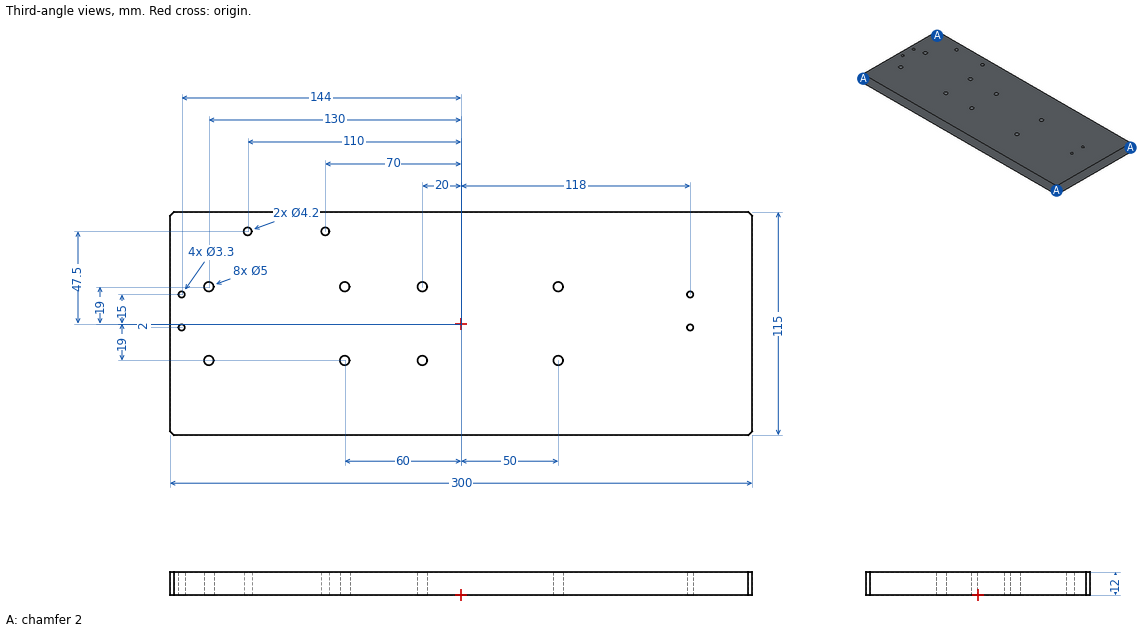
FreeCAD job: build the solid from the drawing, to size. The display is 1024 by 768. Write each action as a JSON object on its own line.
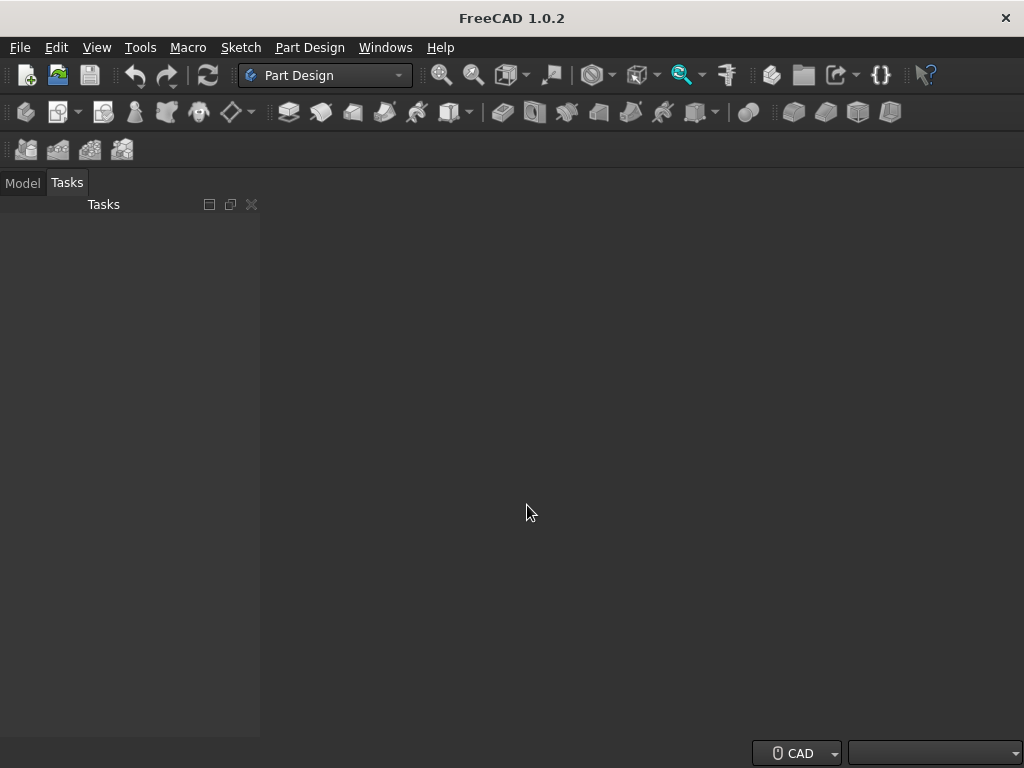
{"action": "left_click", "coordinate": [26, 76]}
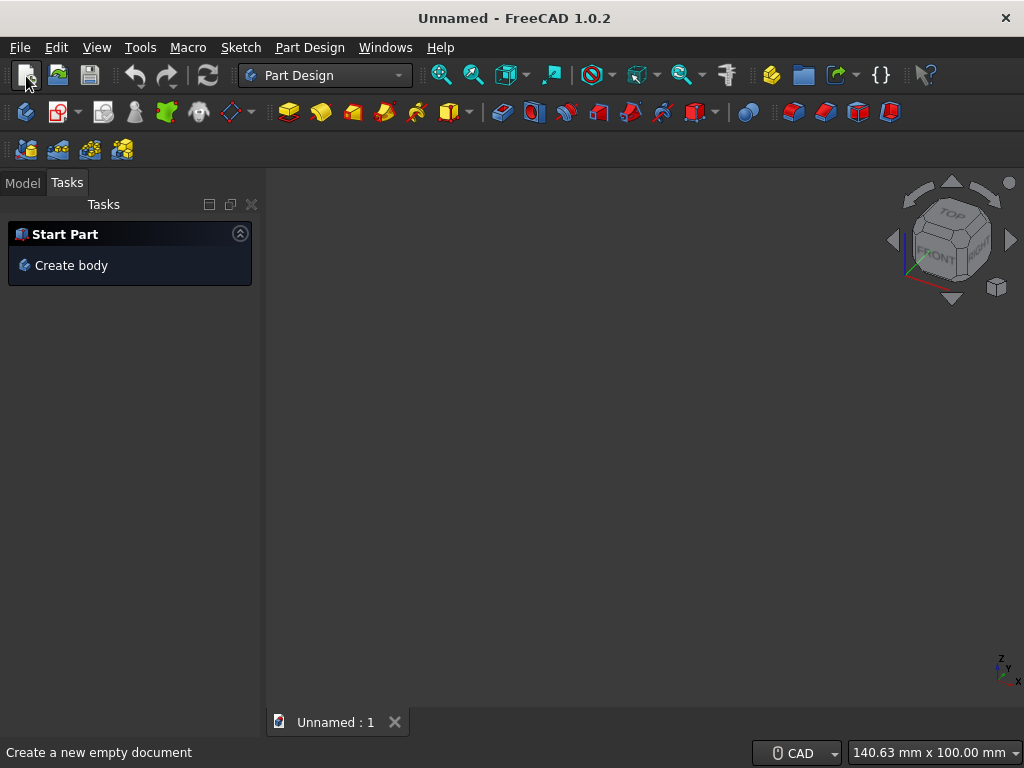
{"action": "left_click", "coordinate": [58, 112]}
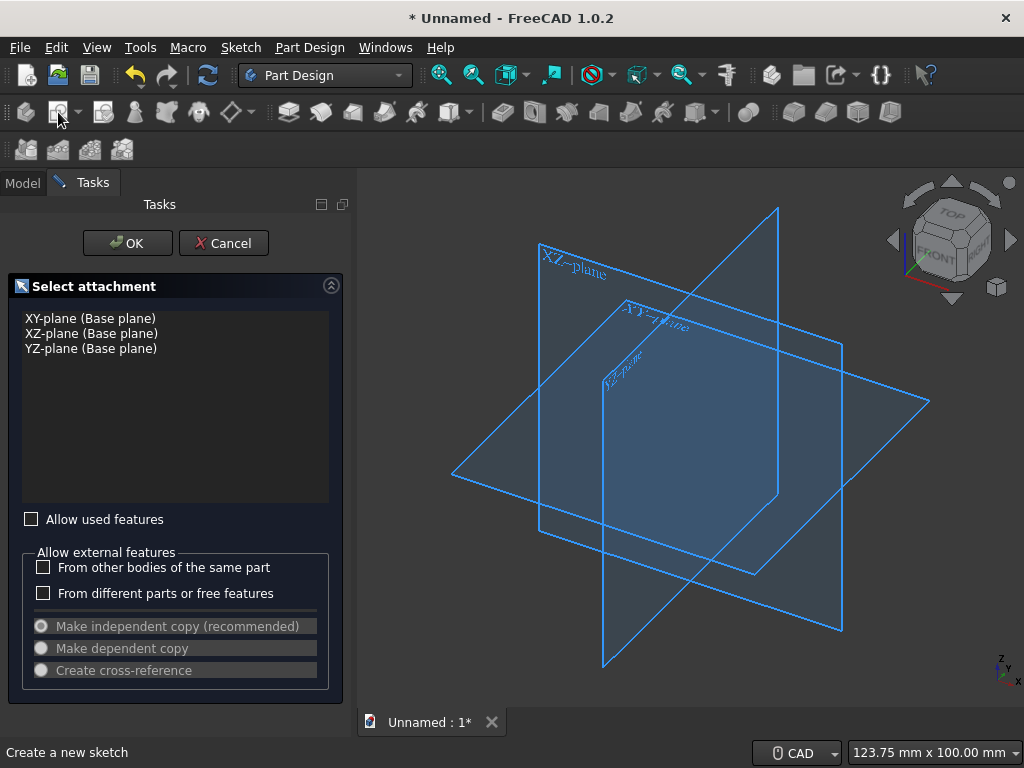
{"action": "left_click", "coordinate": [82, 318]}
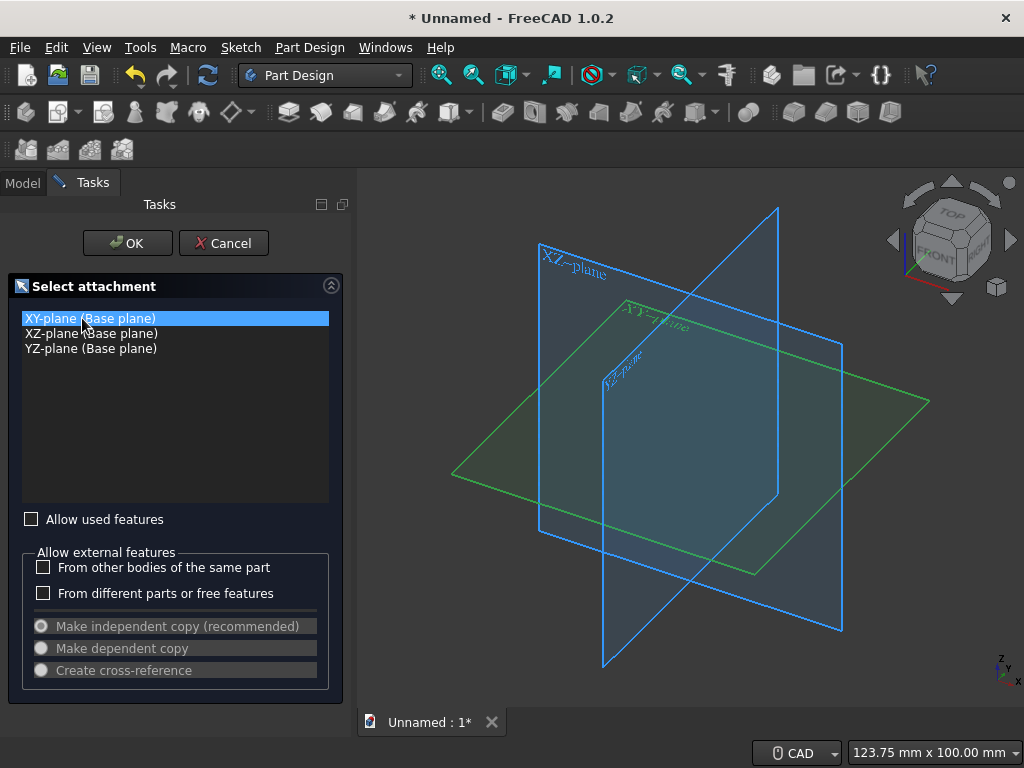
{"action": "left_click", "coordinate": [128, 243]}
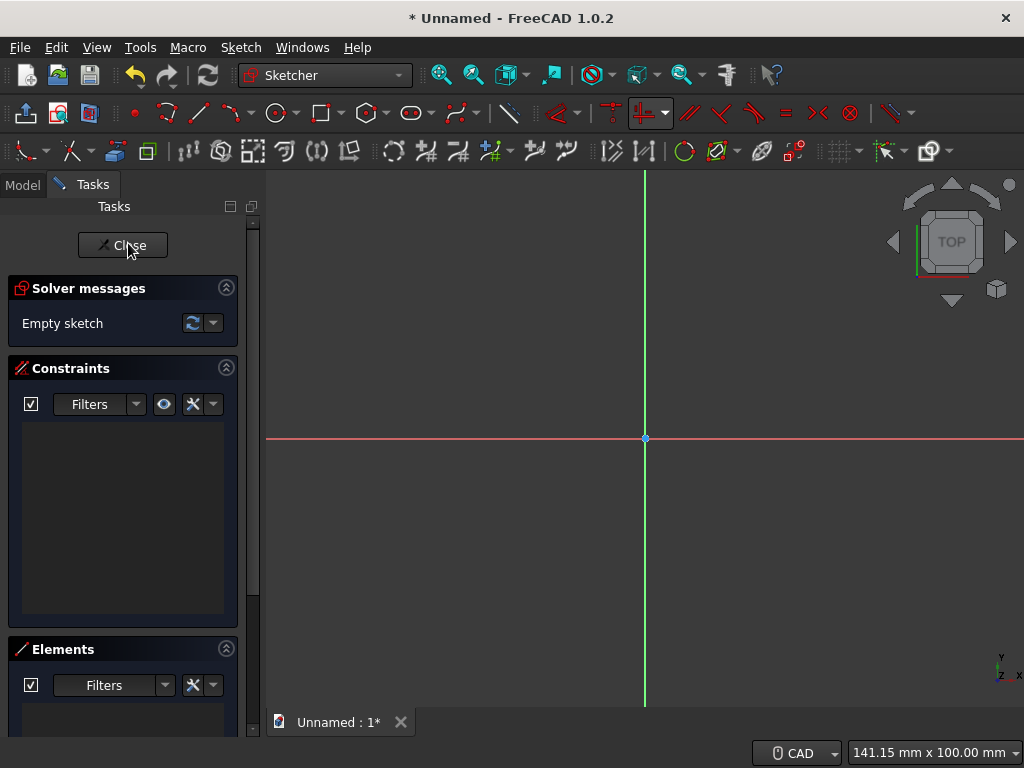
{"action": "scroll", "coordinate": [554, 438], "scroll_direction": "down", "scroll_amount": 7}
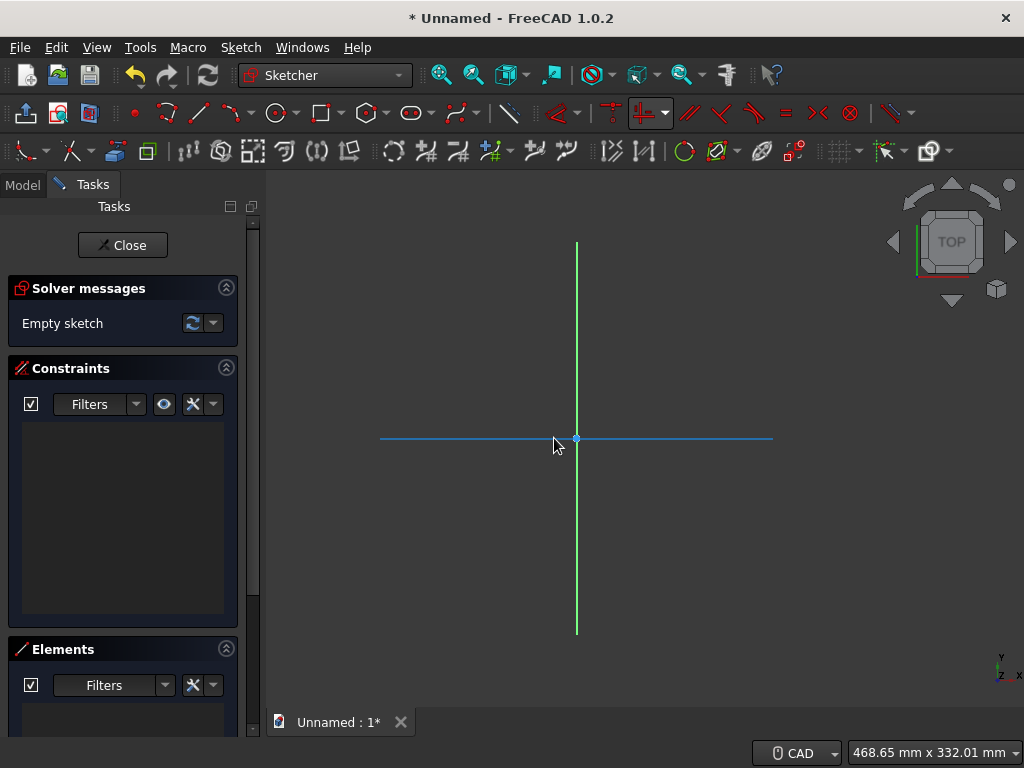
{"action": "key", "text": "g v"}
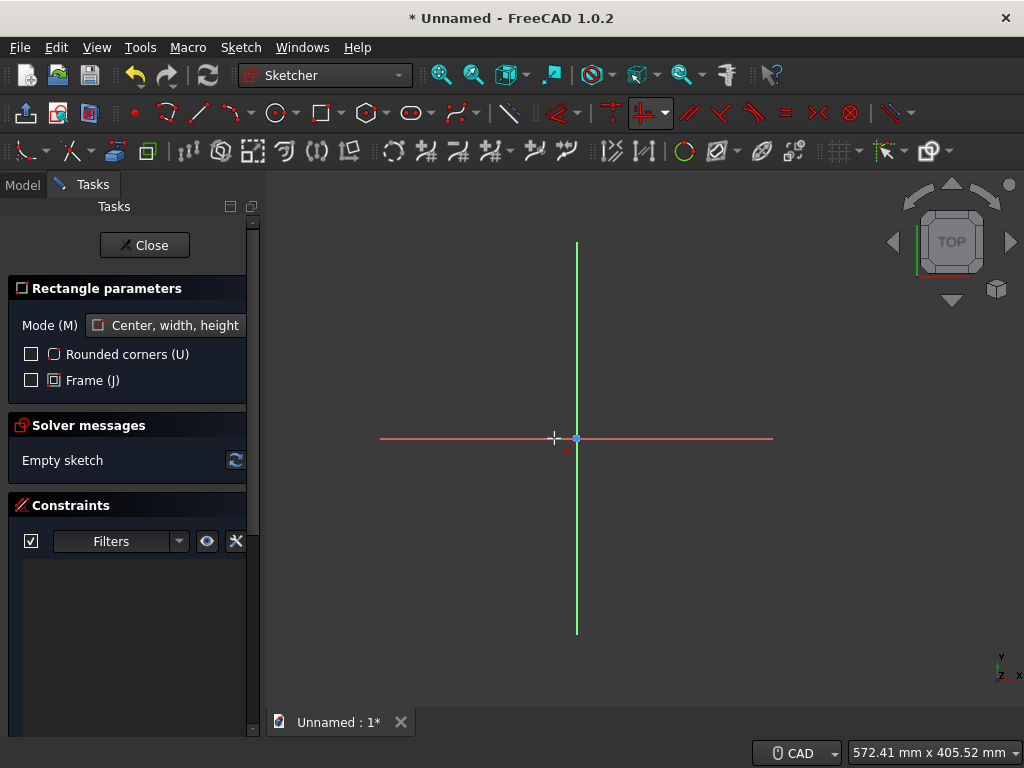
{"action": "left_click", "coordinate": [577, 438]}
{"action": "mouse_move", "coordinate": [775, 362]}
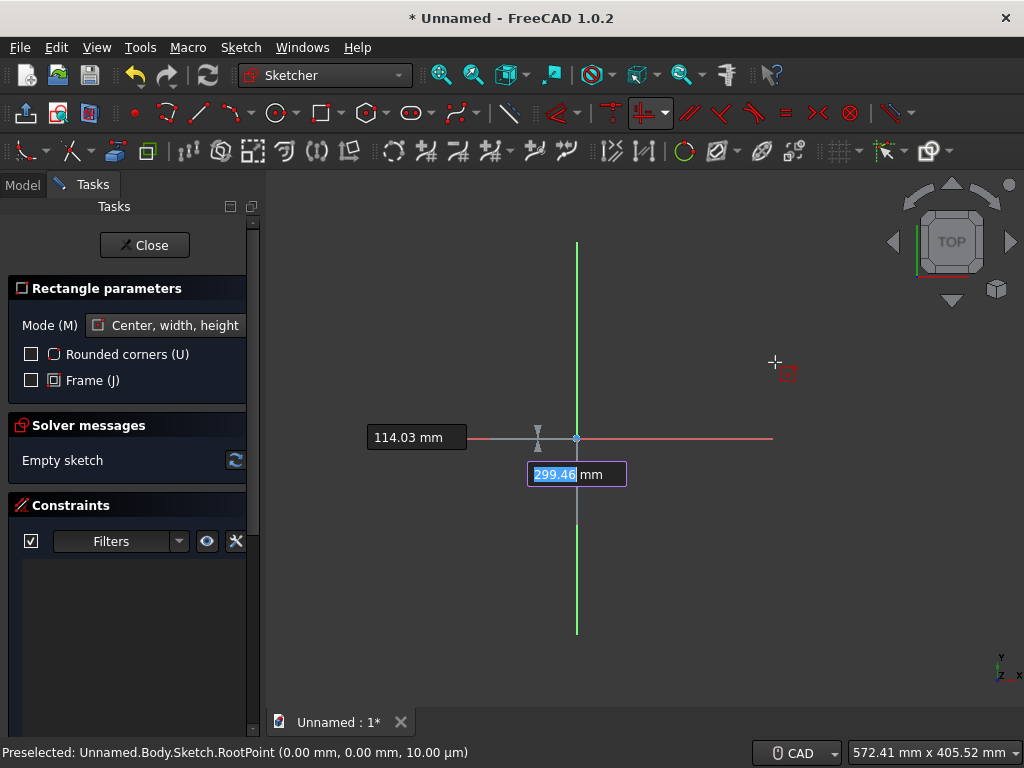
{"action": "type", "text": "300"}
{"action": "key", "text": "Tab"}
{"action": "type", "text": "115"}
{"action": "key", "text": "Return"}
{"action": "key", "text": "Escape"}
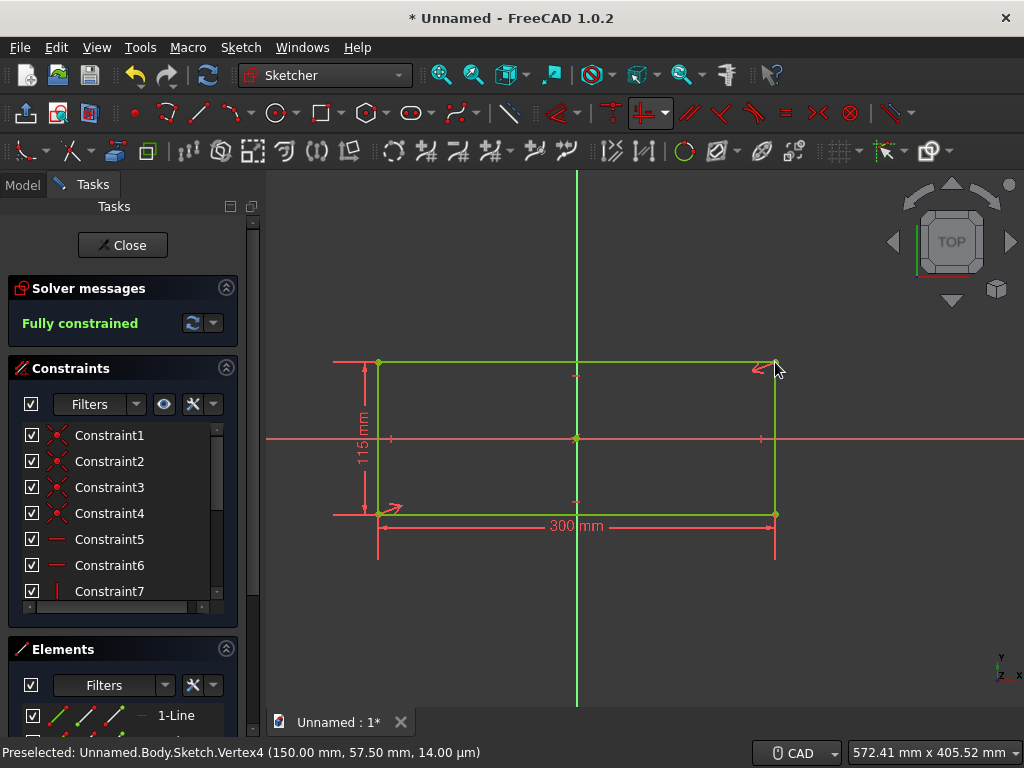
{"action": "left_click", "coordinate": [123, 245]}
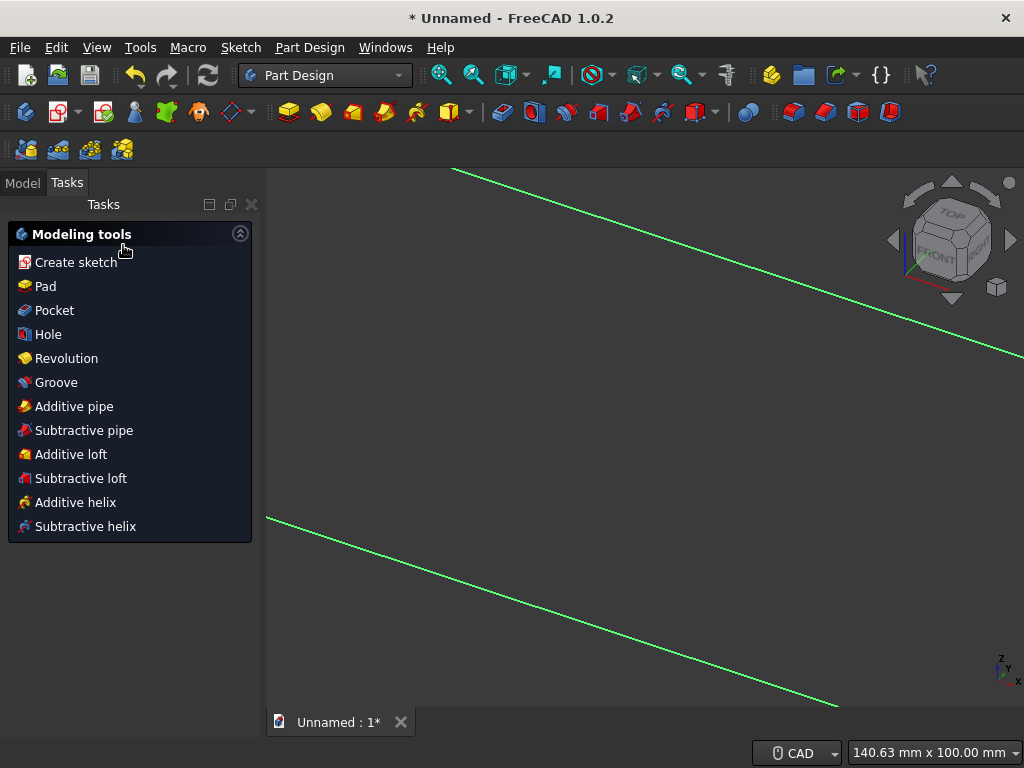
{"action": "left_click", "coordinate": [290, 112]}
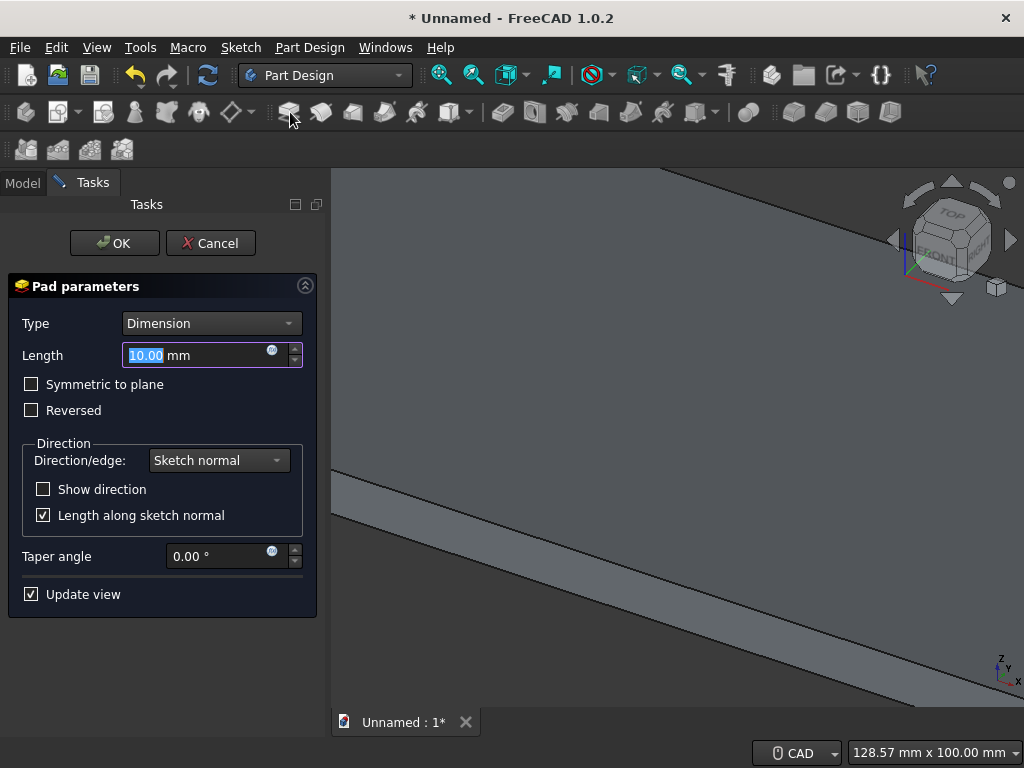
{"action": "type", "text": "12"}
{"action": "key", "text": "Tab"}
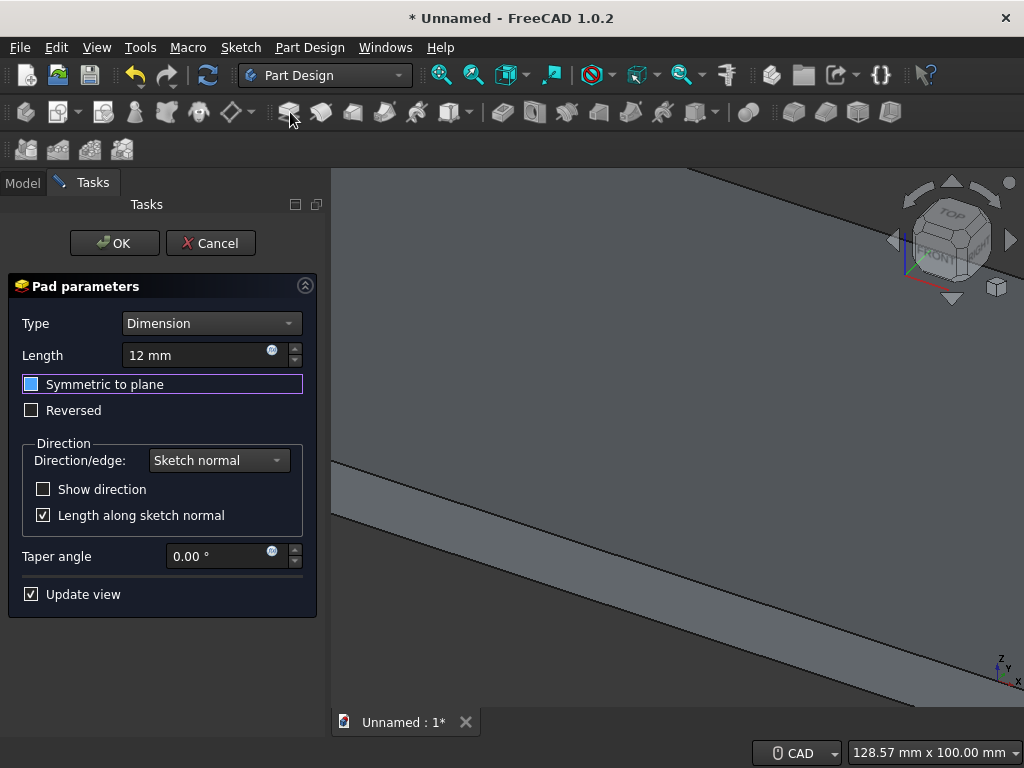
{"action": "left_click", "coordinate": [115, 243]}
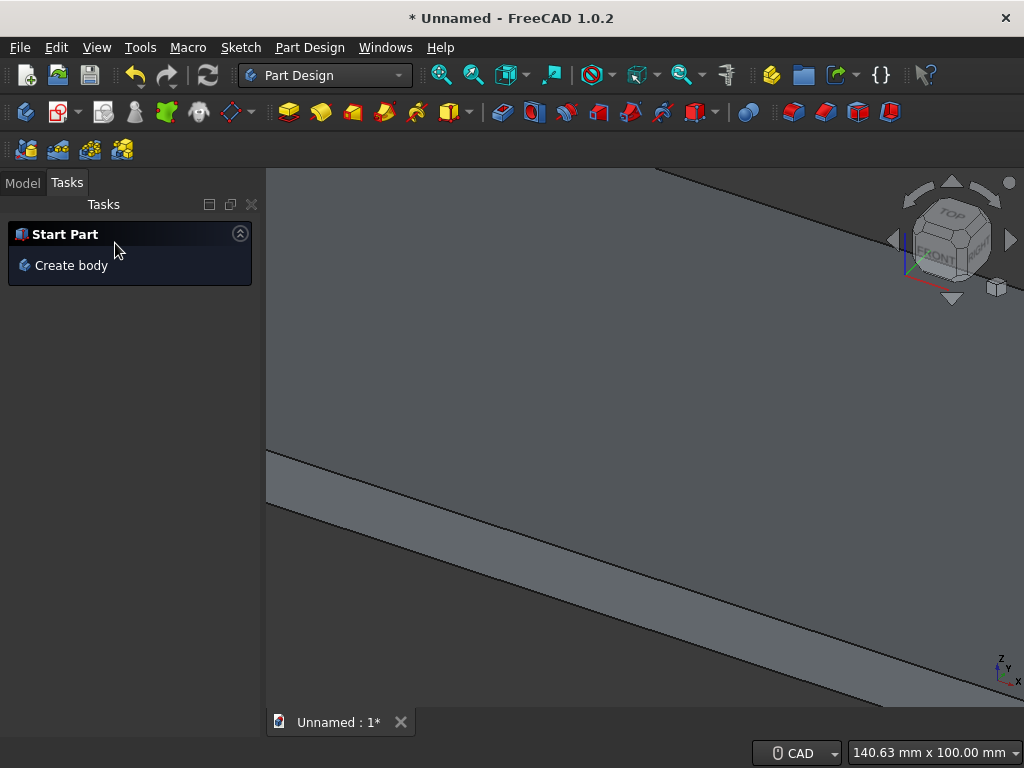
{"action": "key", "text": "v f"}